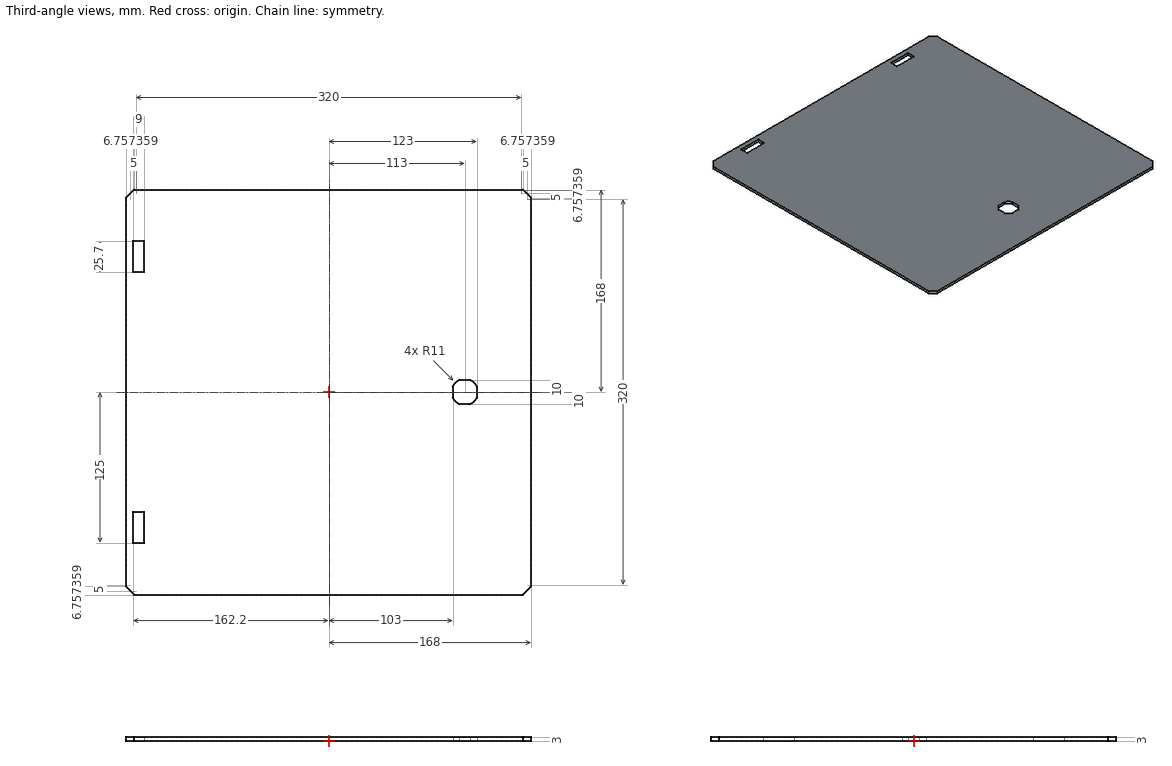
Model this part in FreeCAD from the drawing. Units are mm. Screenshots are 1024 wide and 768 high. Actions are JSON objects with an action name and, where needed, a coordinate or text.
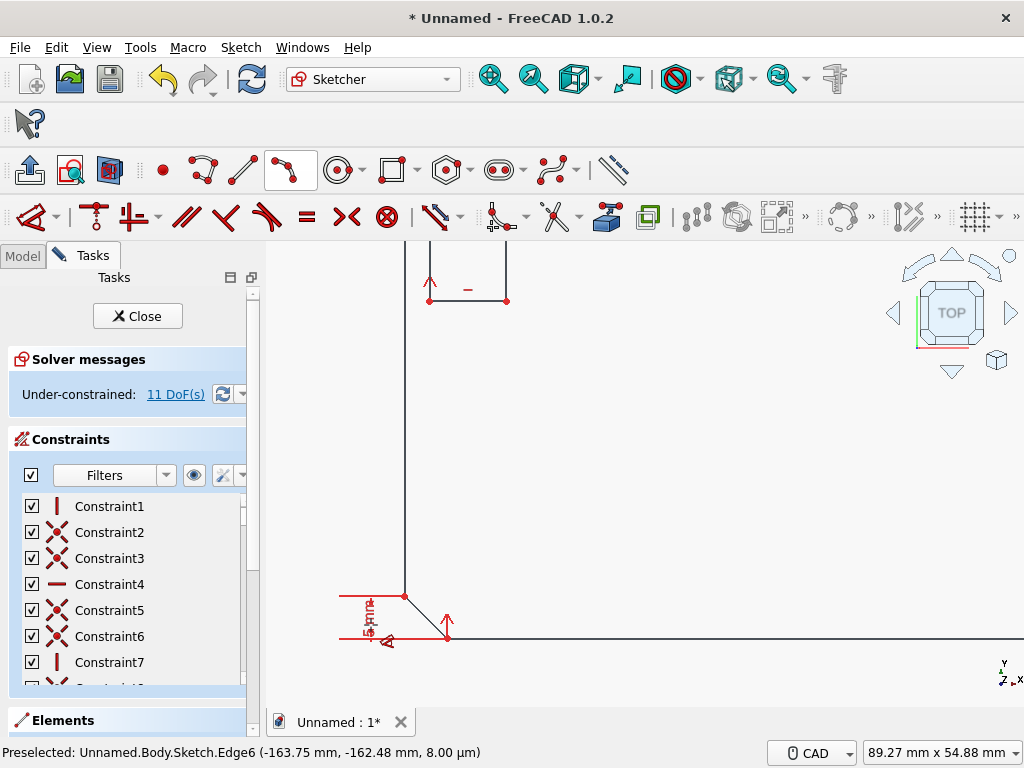
{"action": "scroll", "coordinate": [423, 628], "scroll_direction": "down", "scroll_amount": 11}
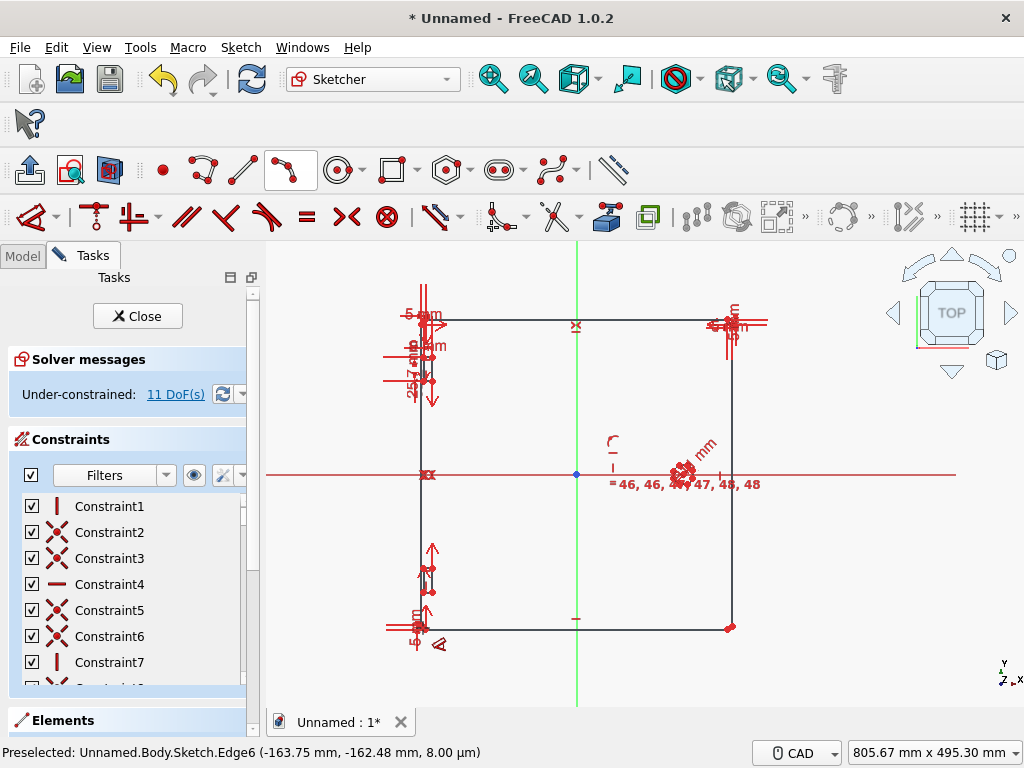
{"action": "scroll", "coordinate": [729, 629], "scroll_direction": "up", "scroll_amount": 11}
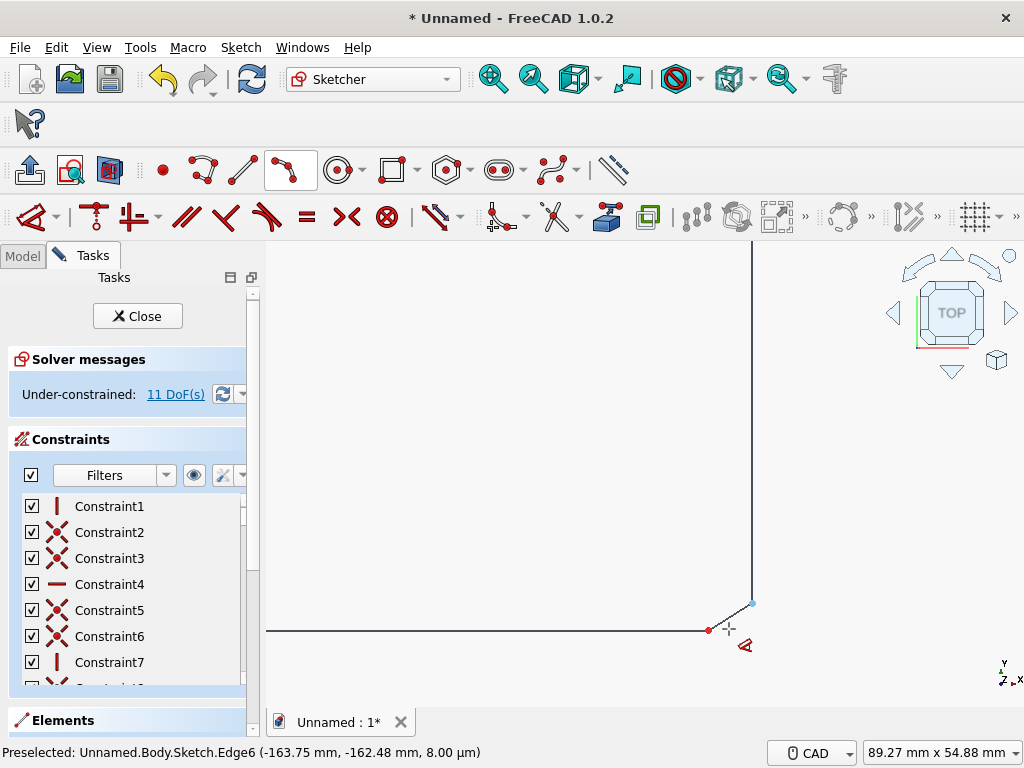
{"action": "left_click", "coordinate": [722, 622]}
{"action": "left_click", "coordinate": [731, 665]}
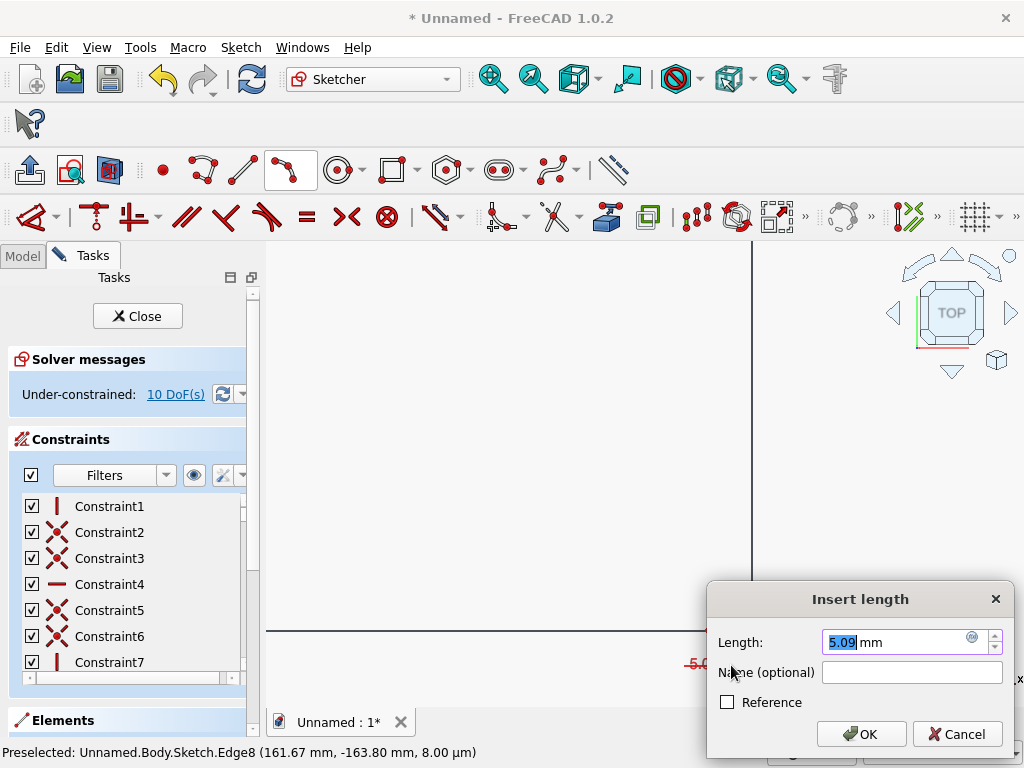
{"action": "type", "text": "5"}
{"action": "key", "text": "Return"}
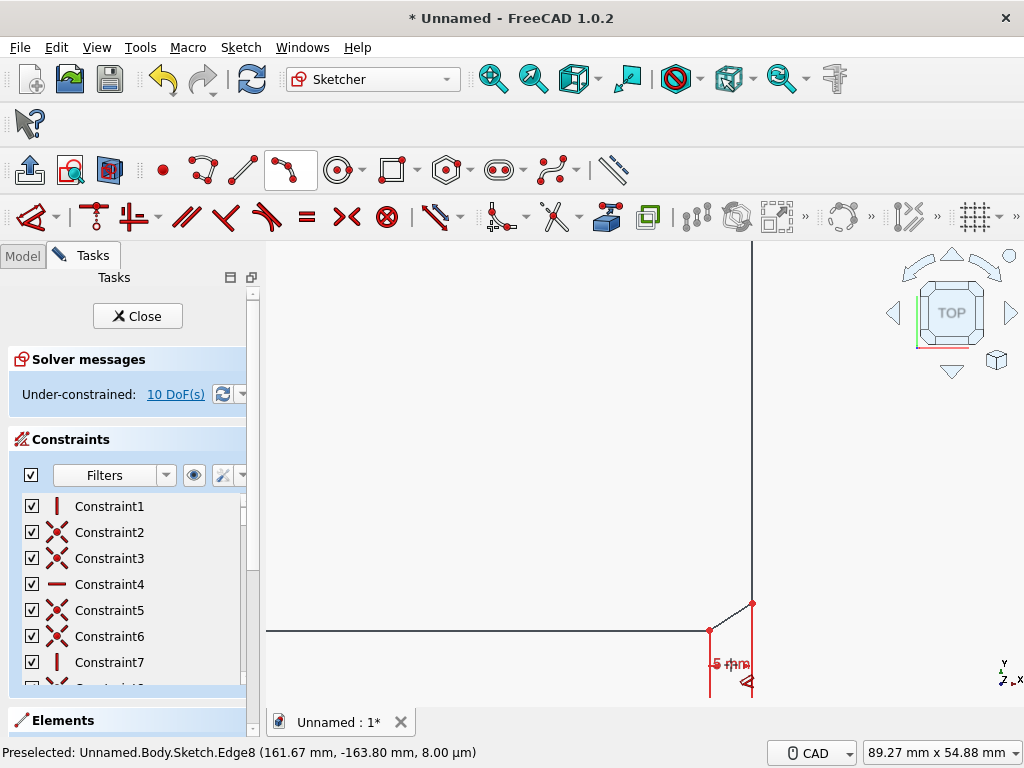
{"action": "left_click", "coordinate": [722, 622]}
{"action": "left_click", "coordinate": [786, 617]}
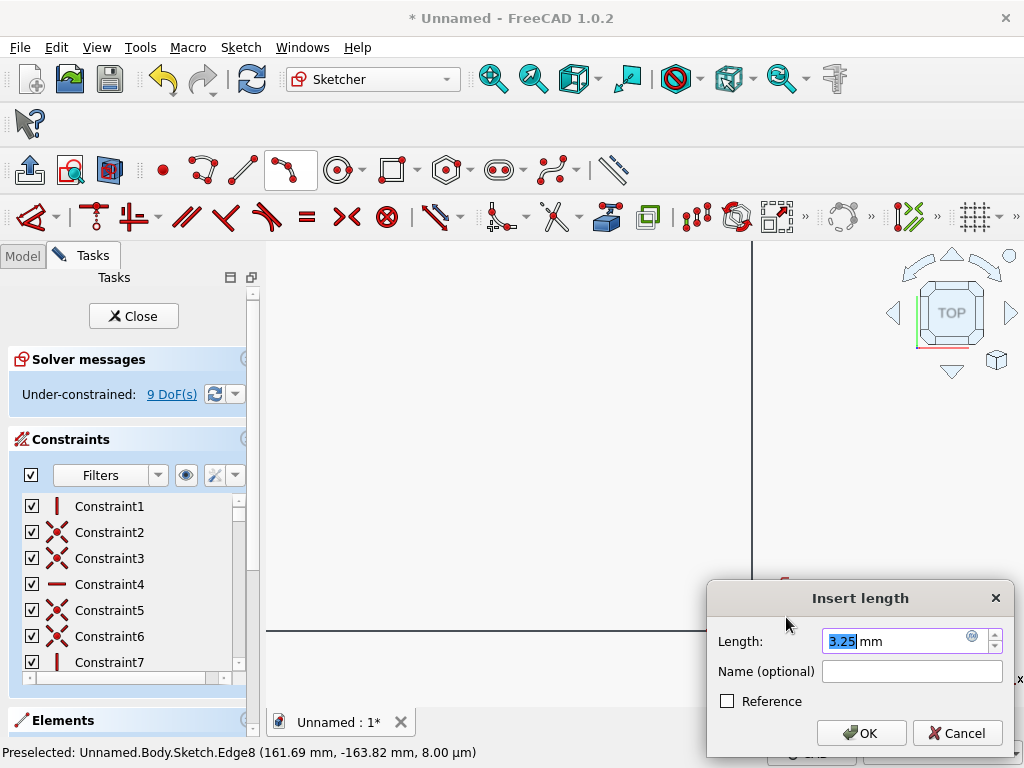
{"action": "type", "text": "5"}
{"action": "key", "text": "Return"}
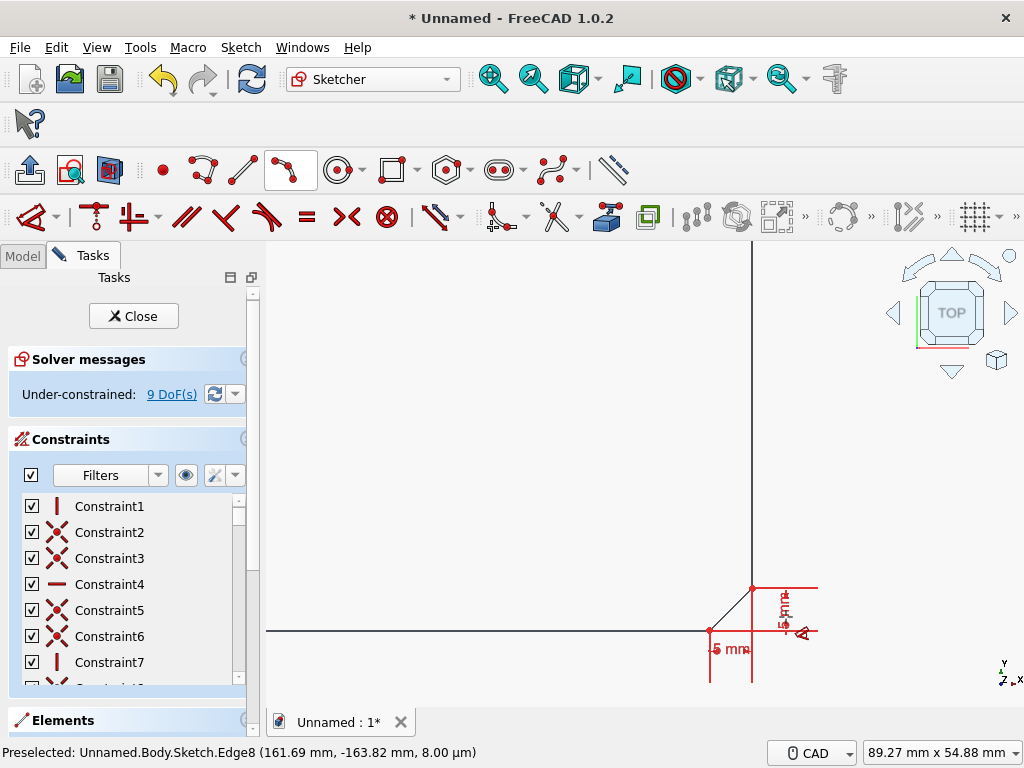
{"action": "scroll", "coordinate": [729, 629], "scroll_direction": "down", "scroll_amount": 11}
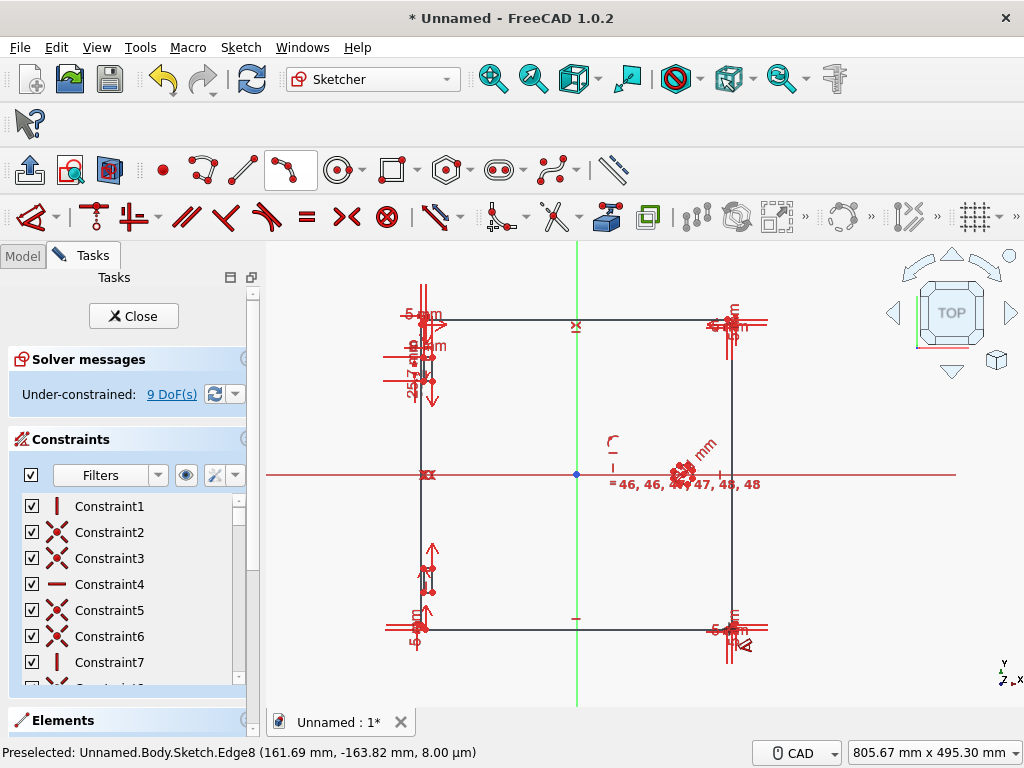
{"action": "left_click", "coordinate": [732, 535]}
{"action": "left_click", "coordinate": [766, 406]}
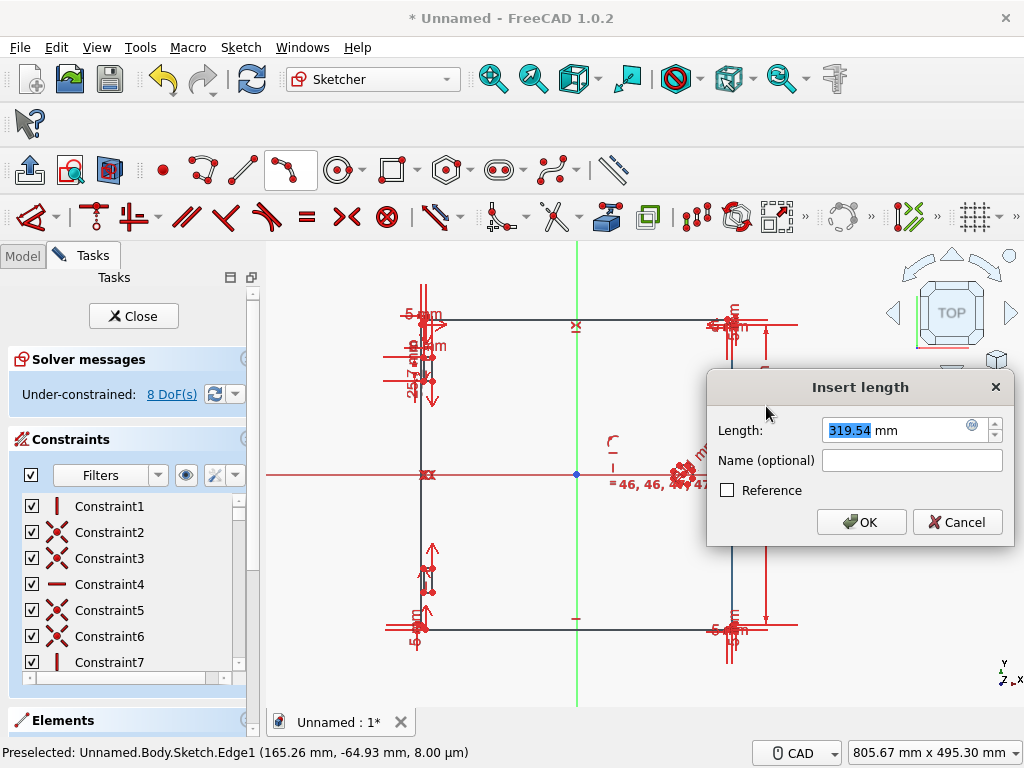
{"action": "type", "text": "320"}
{"action": "key", "text": "Return"}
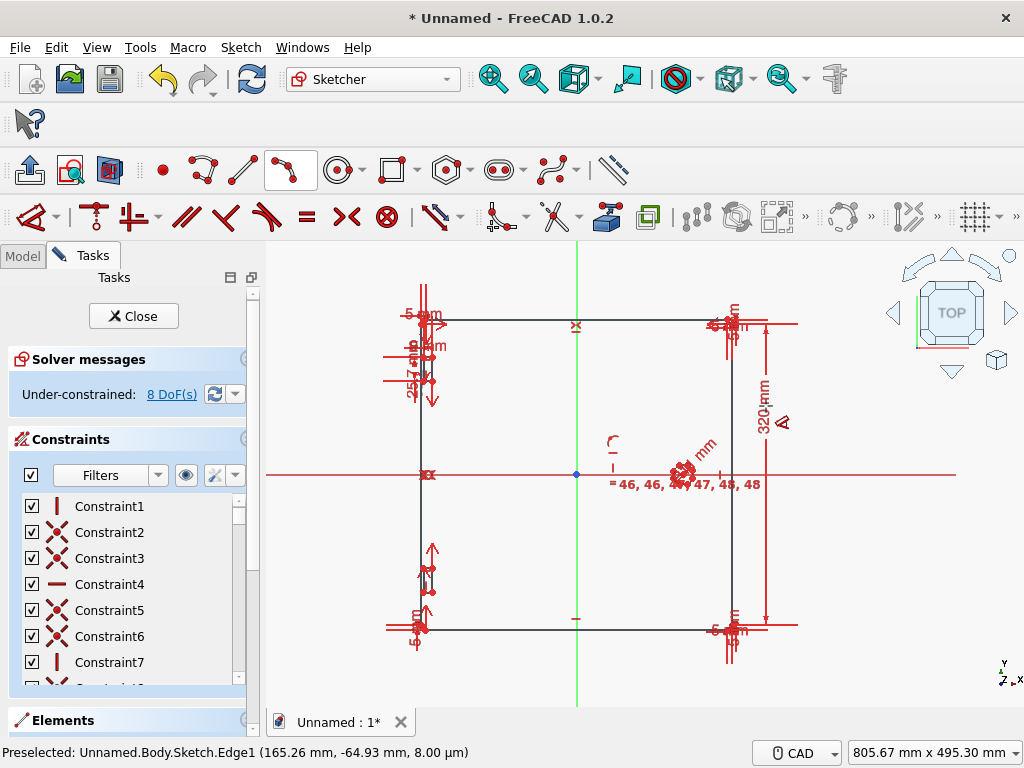
{"action": "left_click", "coordinate": [637, 320]}
{"action": "left_click", "coordinate": [507, 286]}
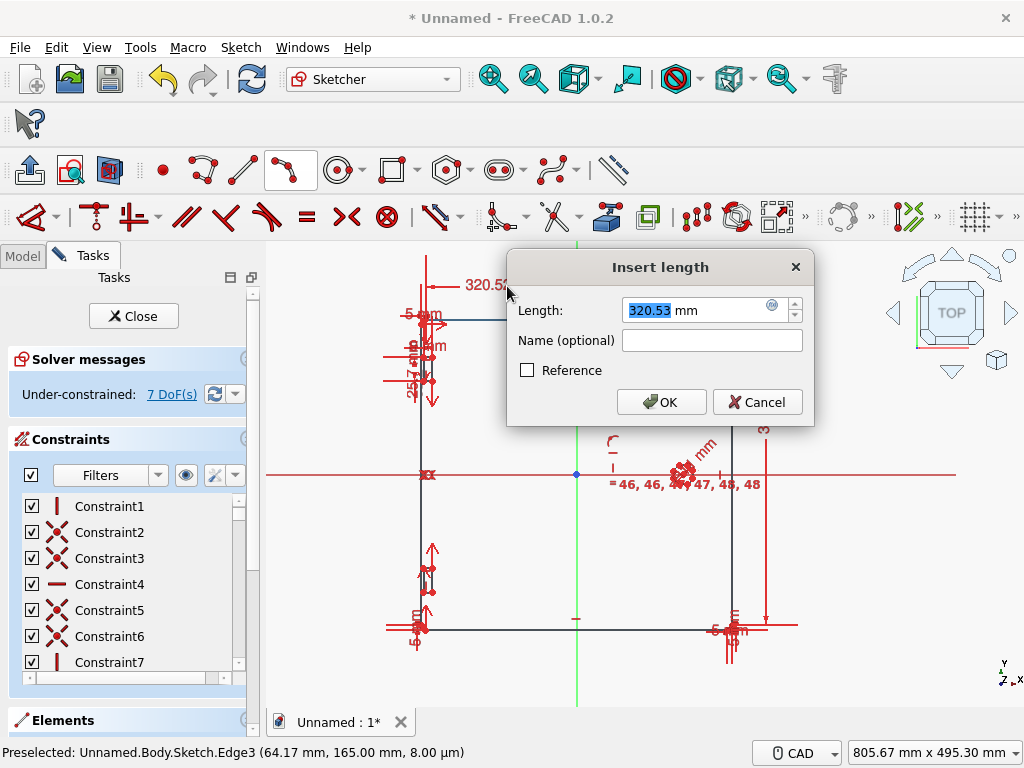
{"action": "type", "text": "320"}
{"action": "key", "text": "Return"}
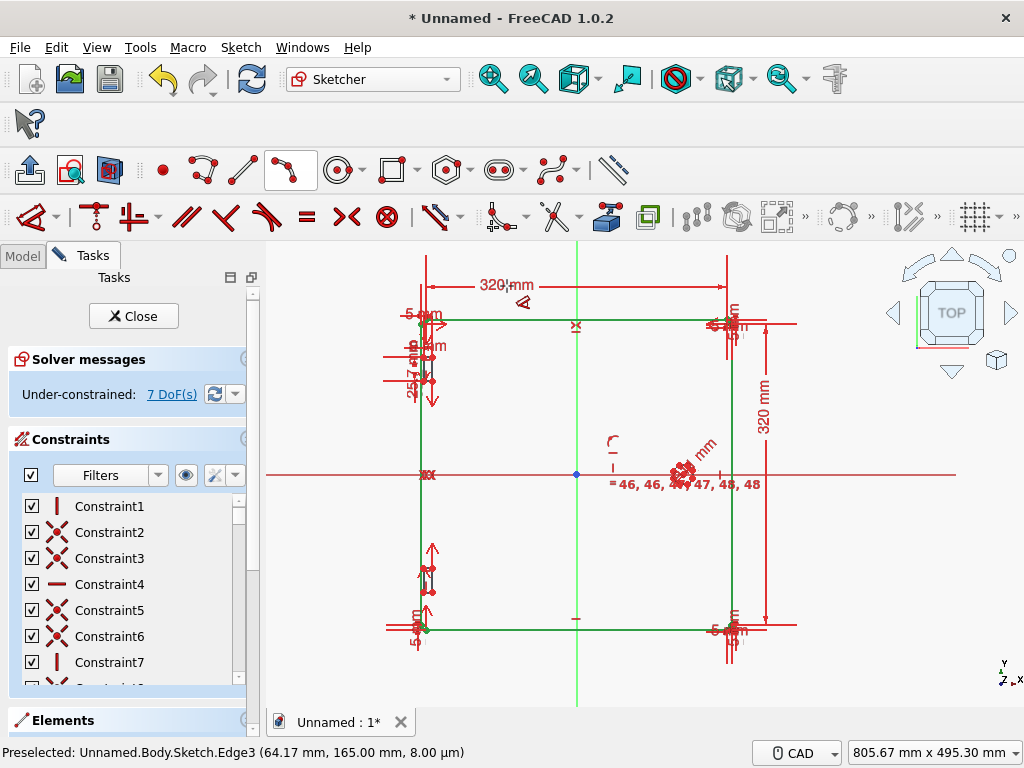
{"action": "scroll", "coordinate": [679, 465], "scroll_direction": "up", "scroll_amount": 8}